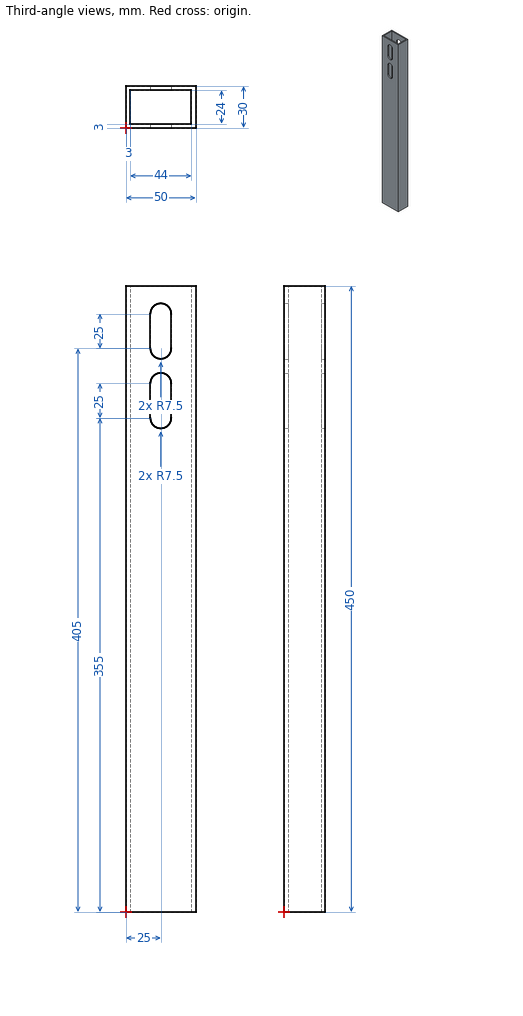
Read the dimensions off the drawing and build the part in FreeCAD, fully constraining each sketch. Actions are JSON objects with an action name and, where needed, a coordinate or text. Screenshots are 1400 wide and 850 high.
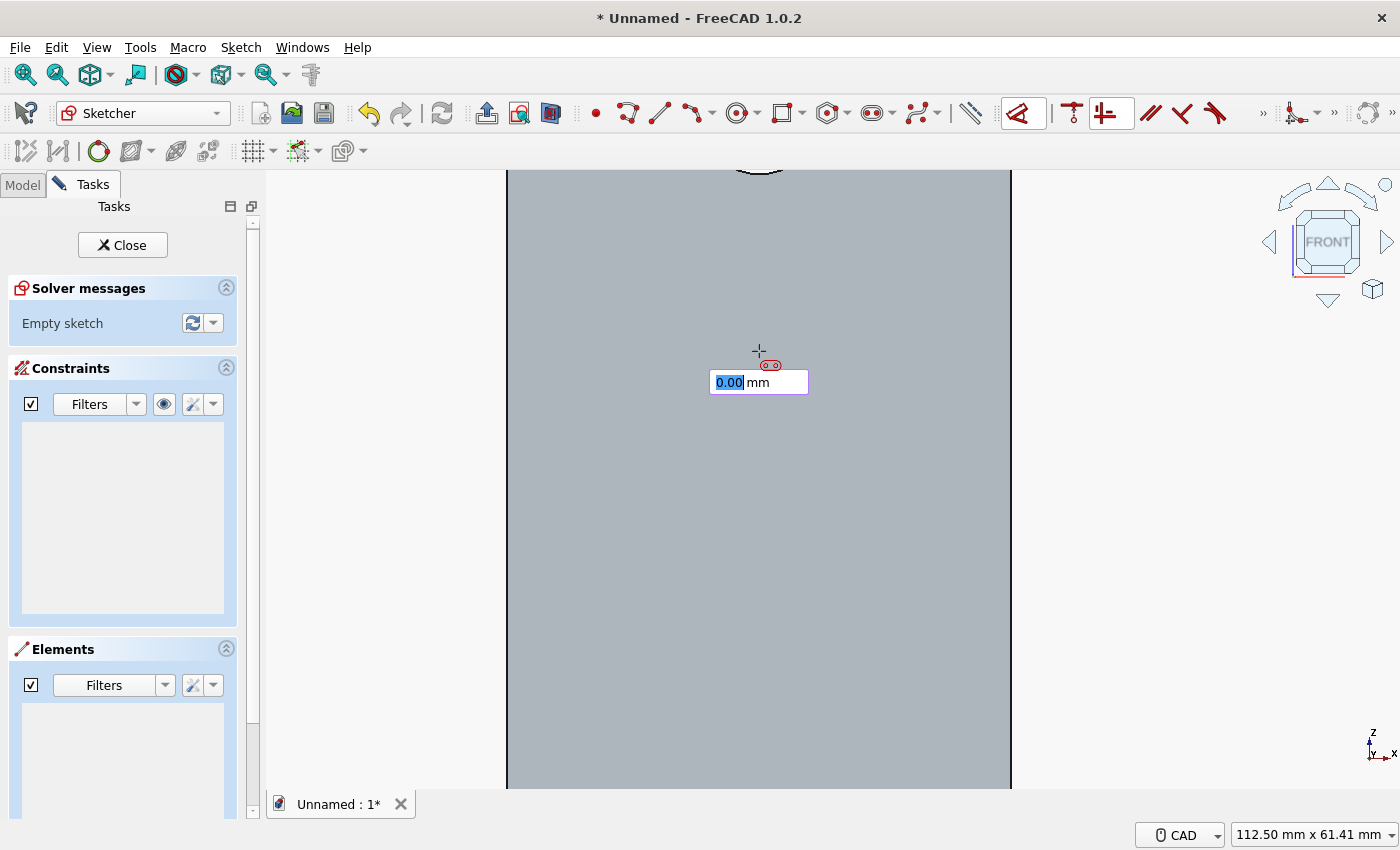
{"action": "left_click", "coordinate": [684, 477]}
{"action": "key", "text": "Escape"}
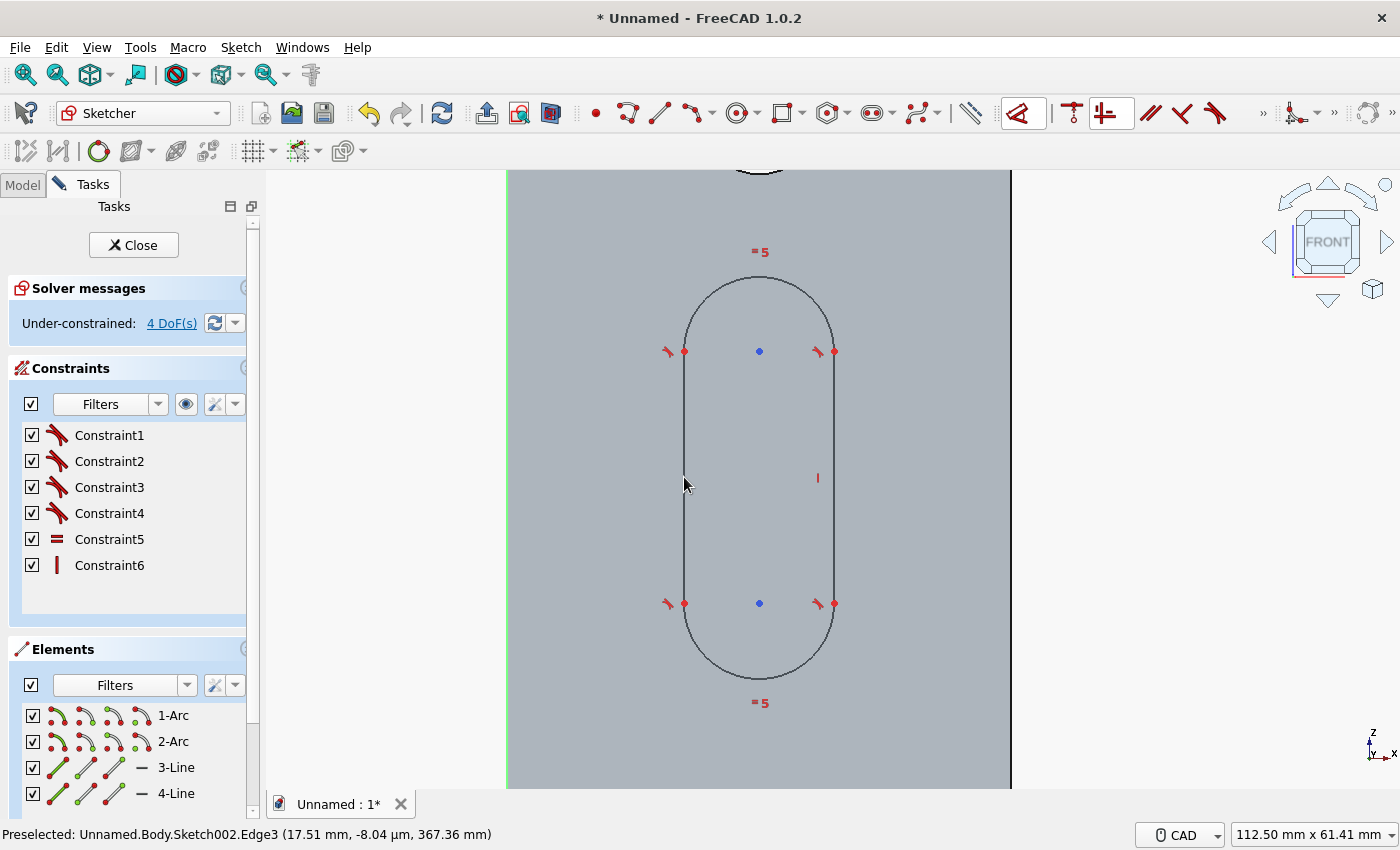
{"action": "left_click", "coordinate": [715, 665]}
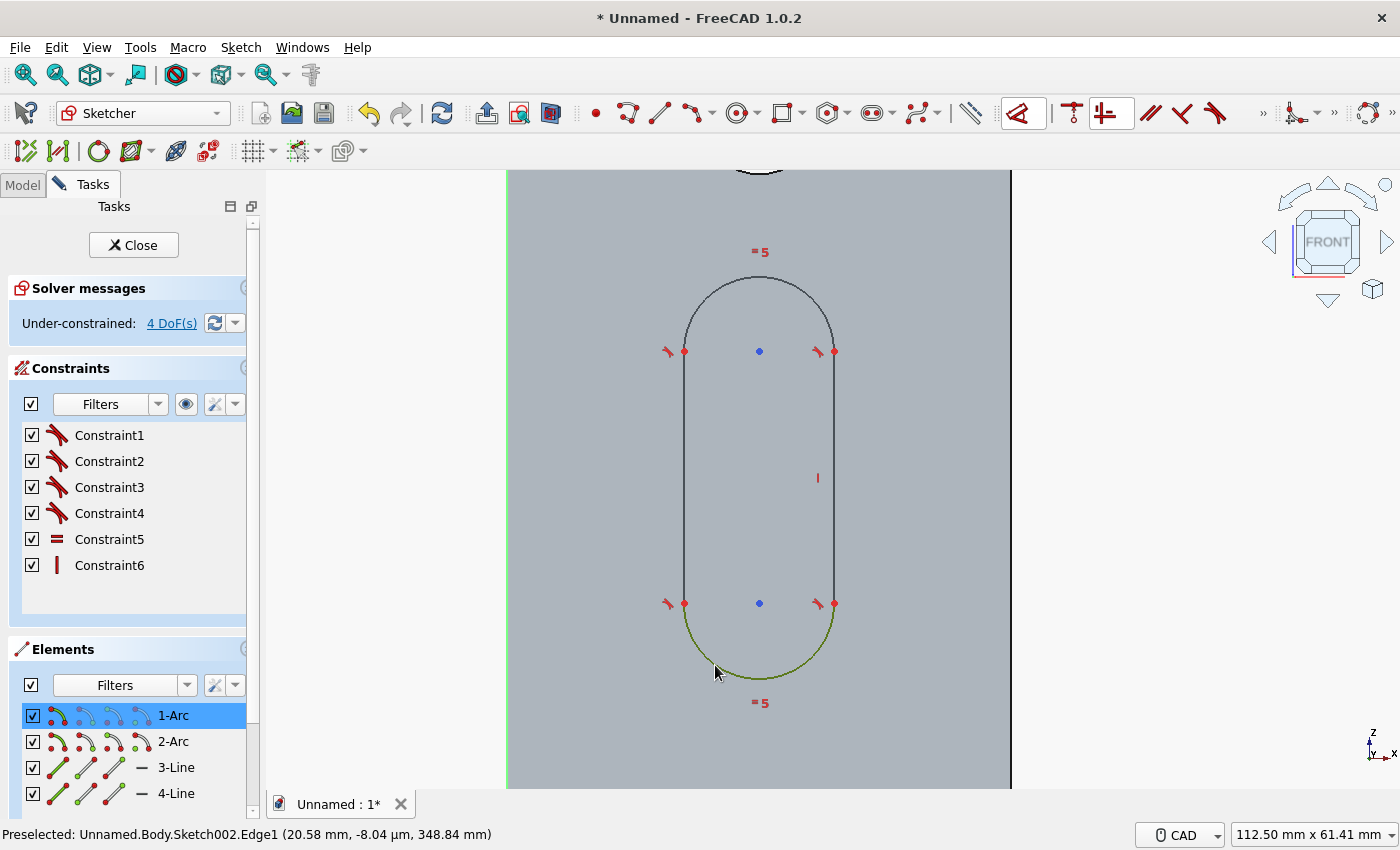
{"action": "left_click", "coordinate": [1040, 114]}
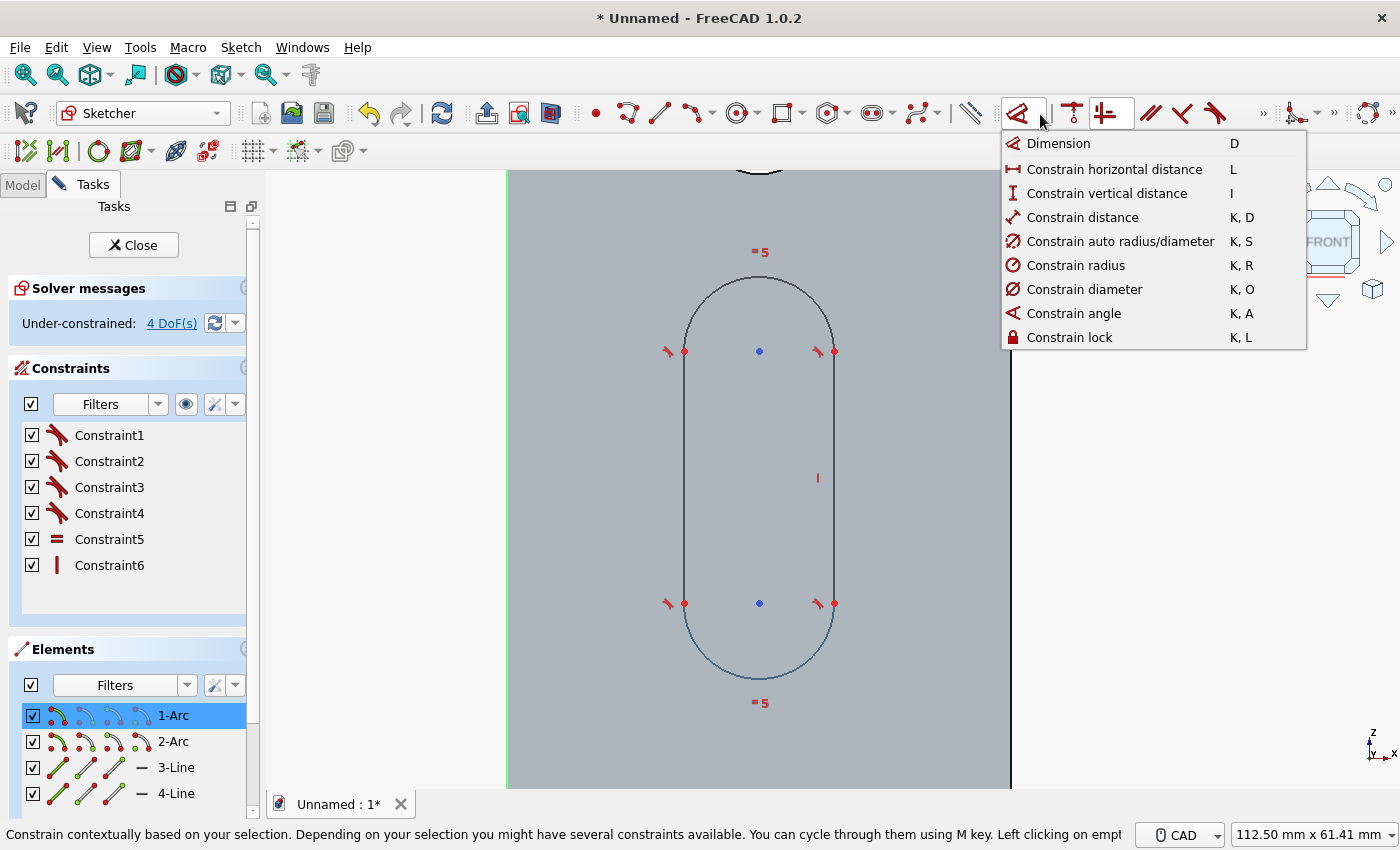
{"action": "left_click", "coordinate": [1154, 265]}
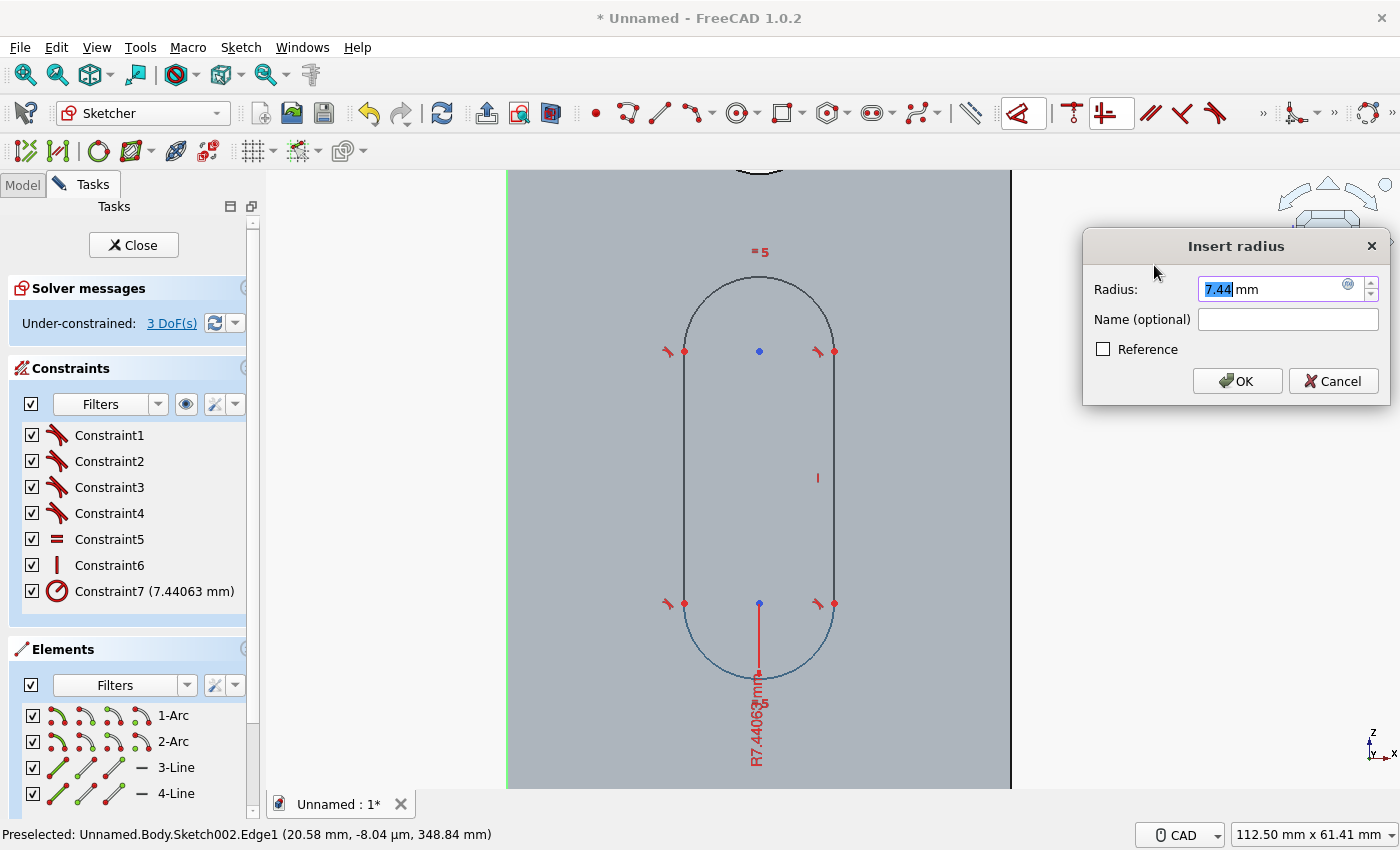
{"action": "type", "text": "7.5"}
{"action": "key", "text": "Return"}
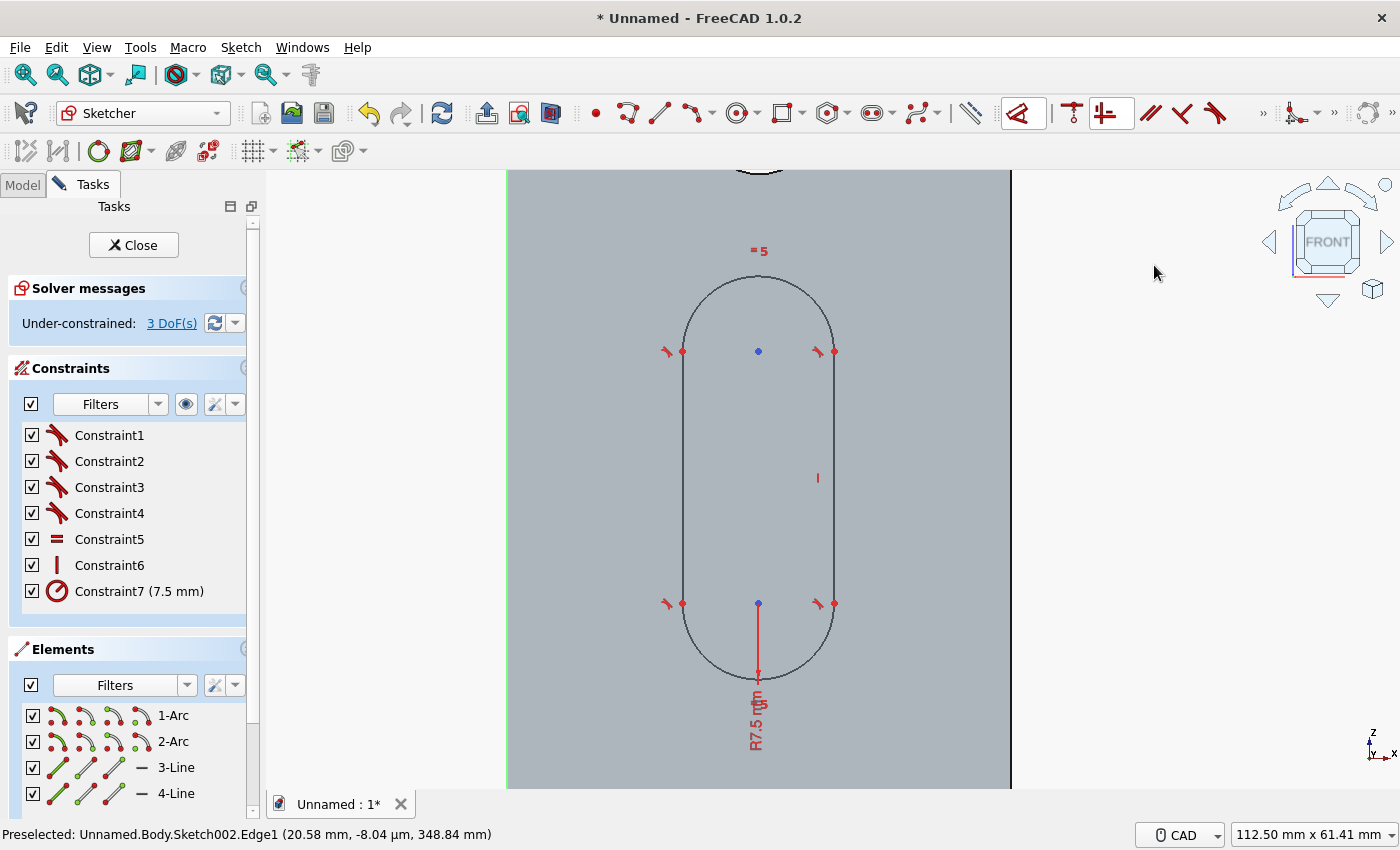
{"action": "left_click", "coordinate": [683, 528]}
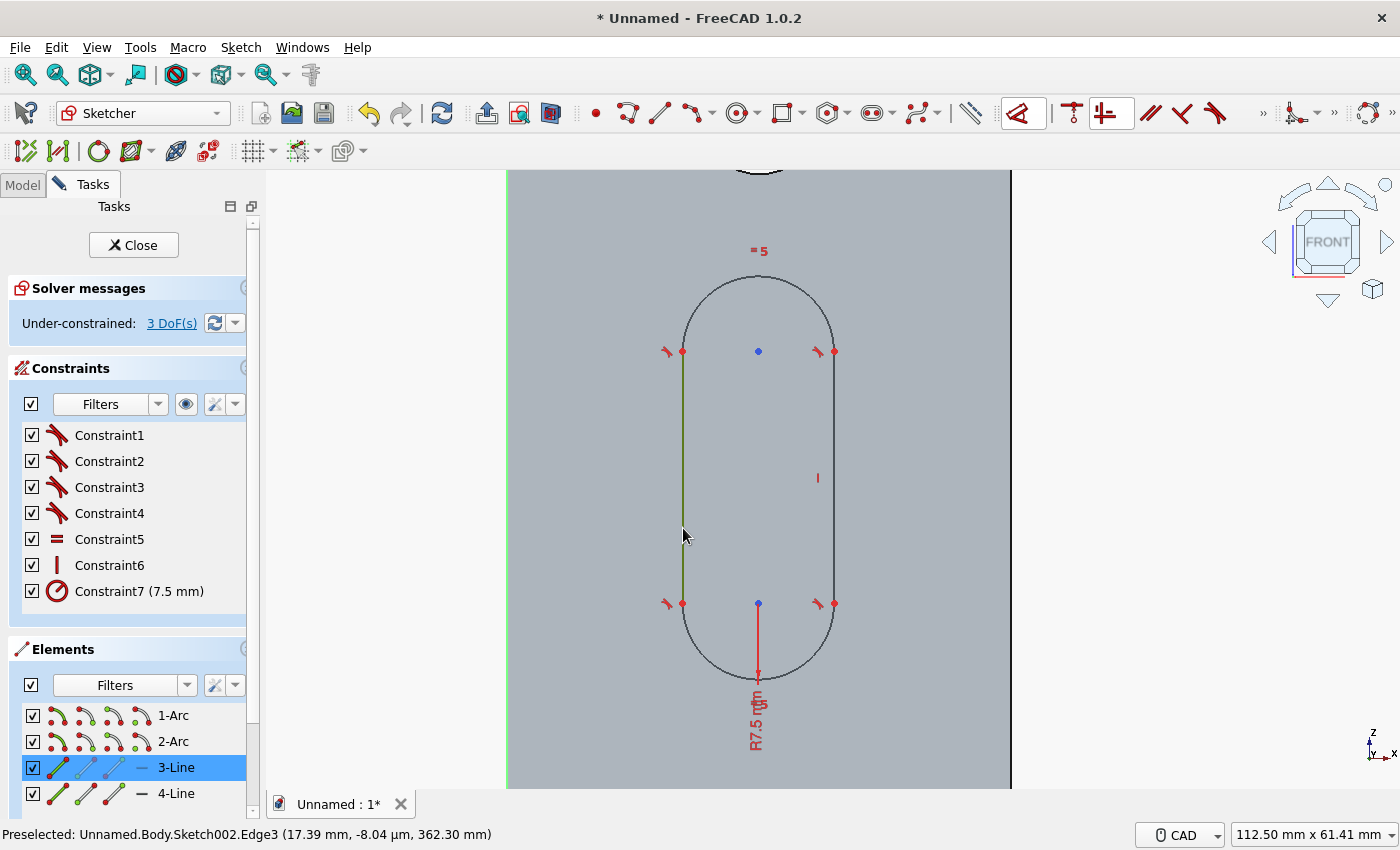
{"action": "left_click", "coordinate": [1040, 114]}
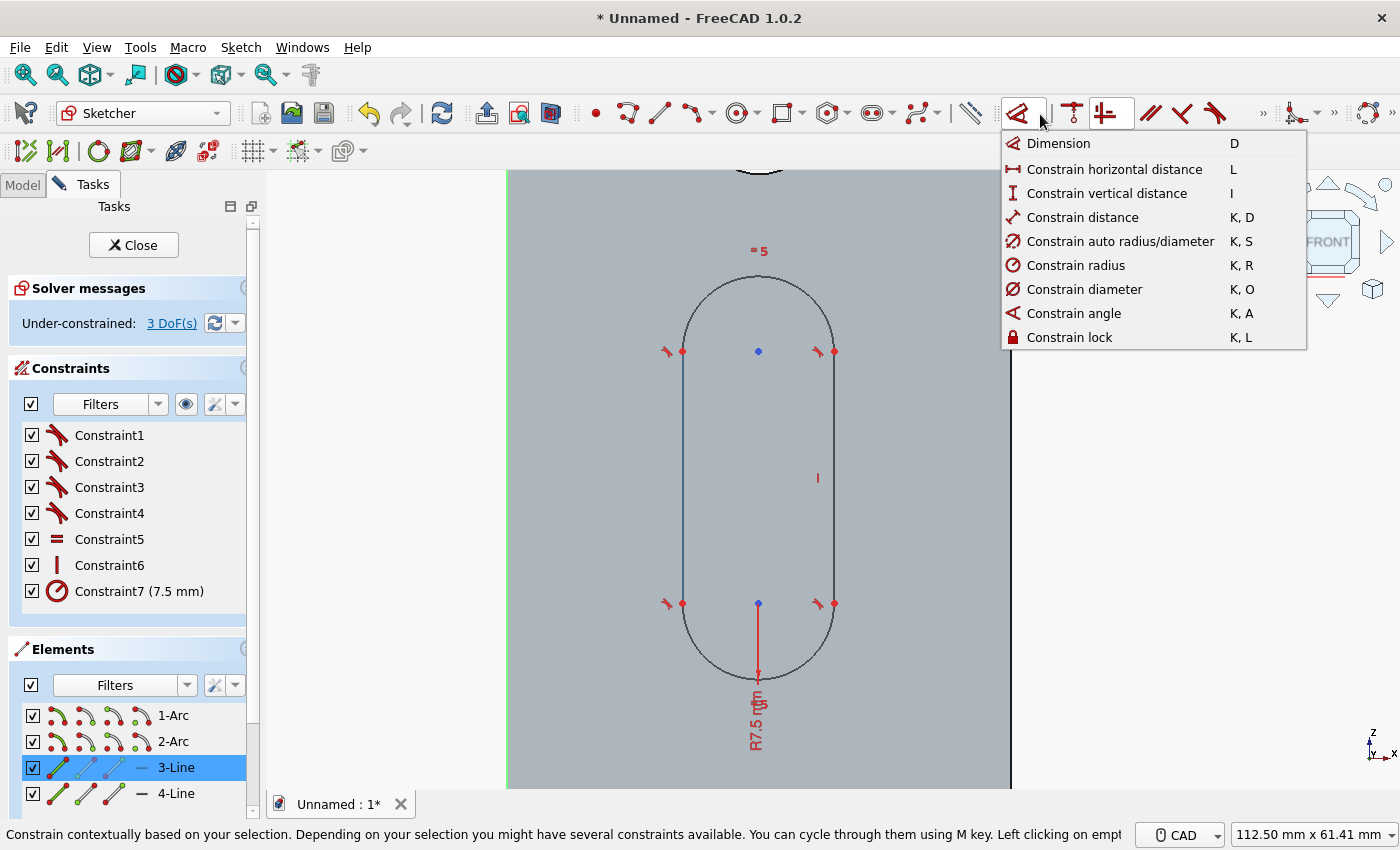
{"action": "left_click", "coordinate": [1154, 193]}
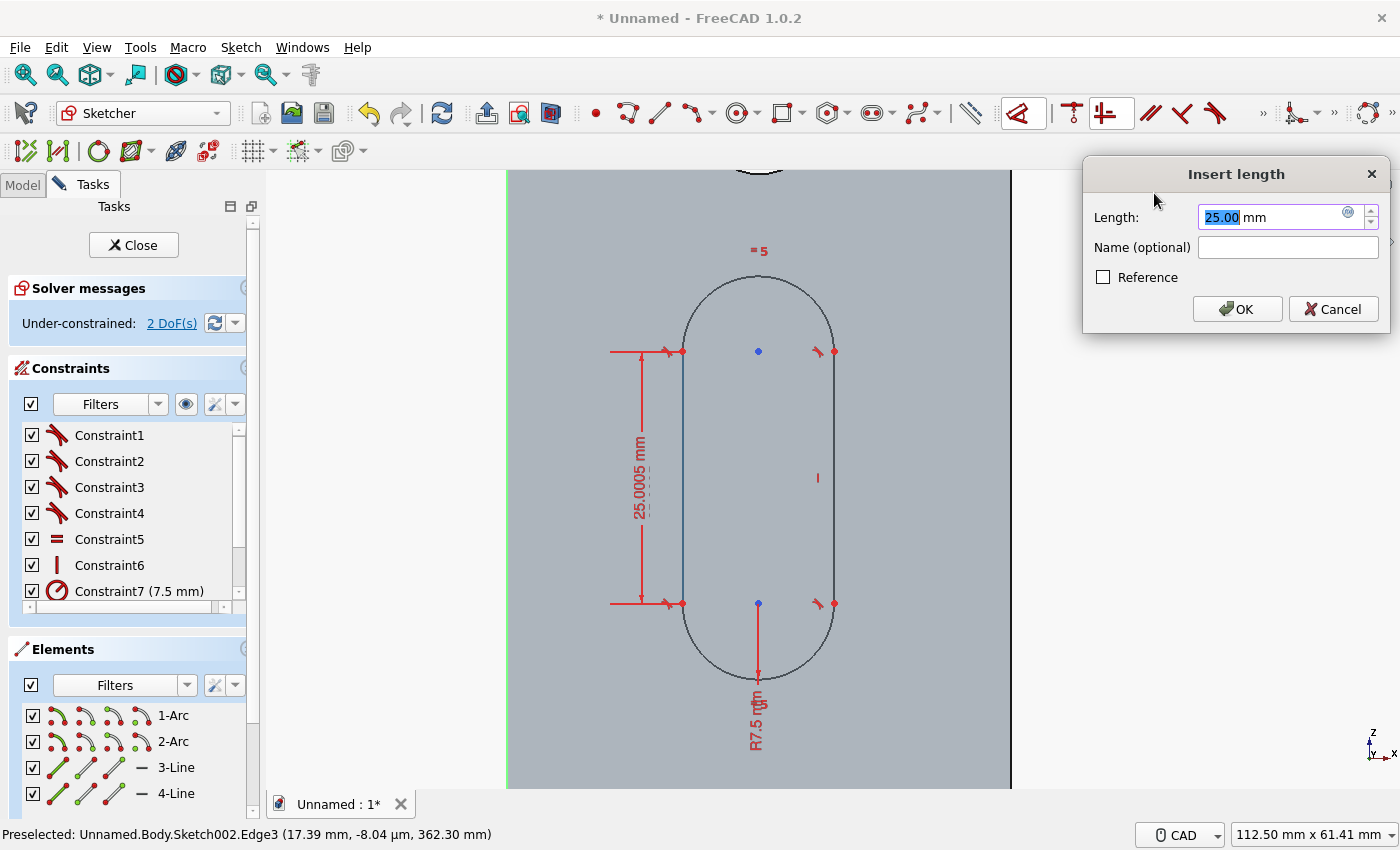
{"action": "type", "text": "25"}
{"action": "key", "text": "Return"}